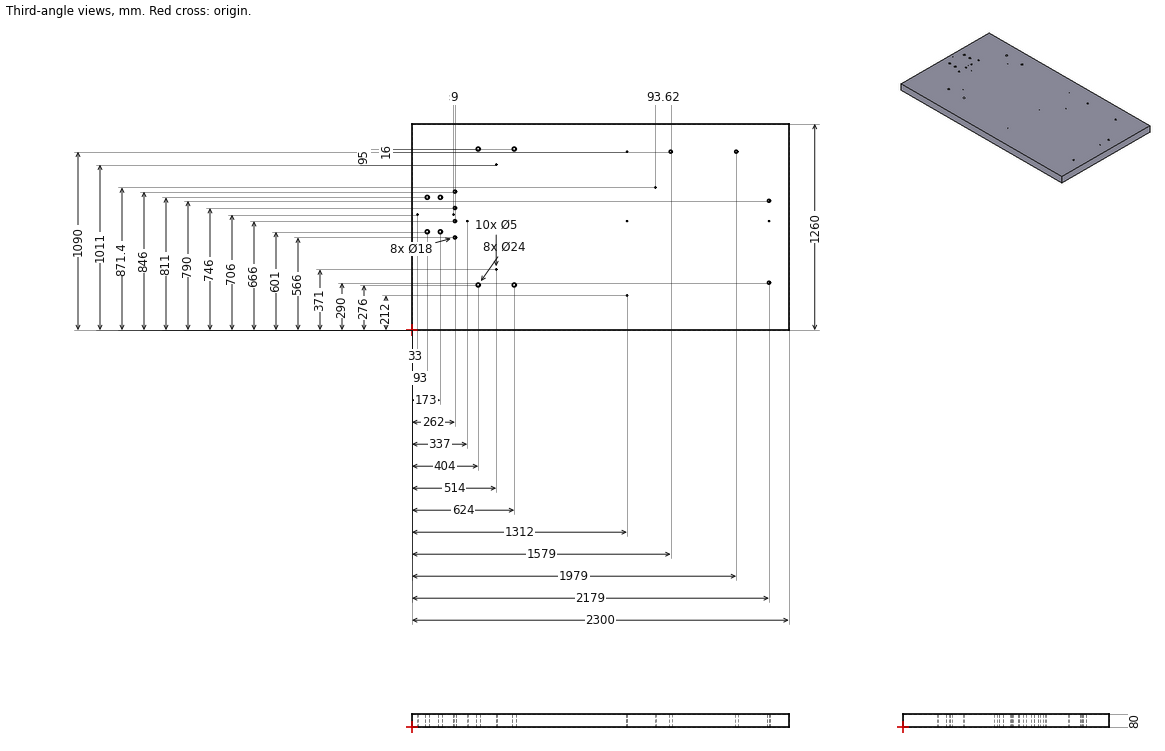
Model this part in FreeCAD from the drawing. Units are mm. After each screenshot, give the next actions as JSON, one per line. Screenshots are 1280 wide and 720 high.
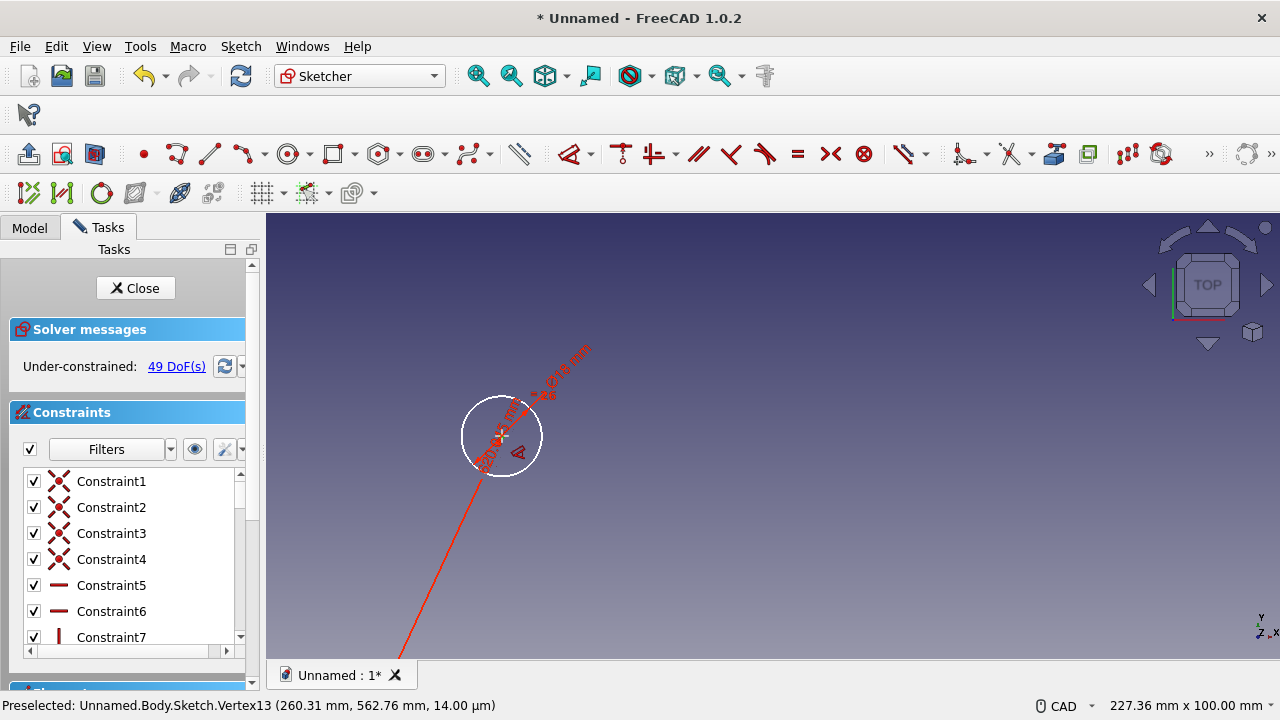
{"action": "scroll", "coordinate": [507, 452], "scroll_direction": "down", "scroll_amount": 15}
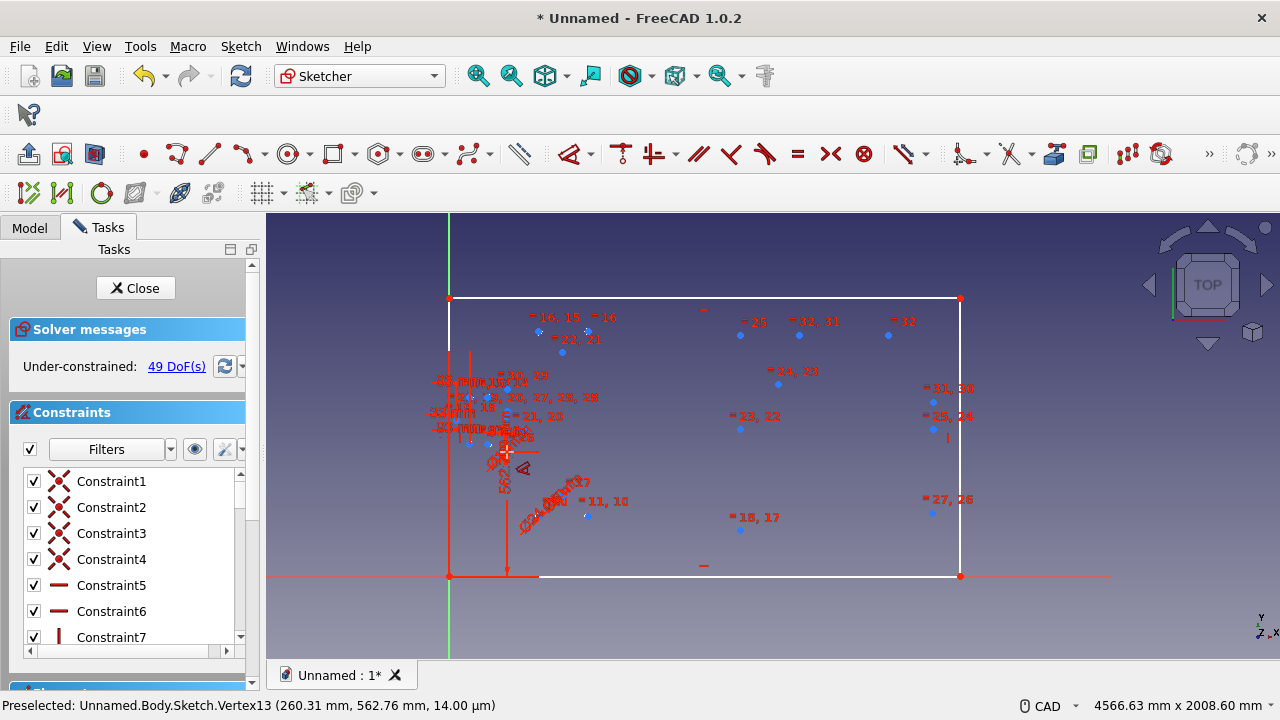
{"action": "scroll", "coordinate": [505, 420], "scroll_direction": "up", "scroll_amount": 15}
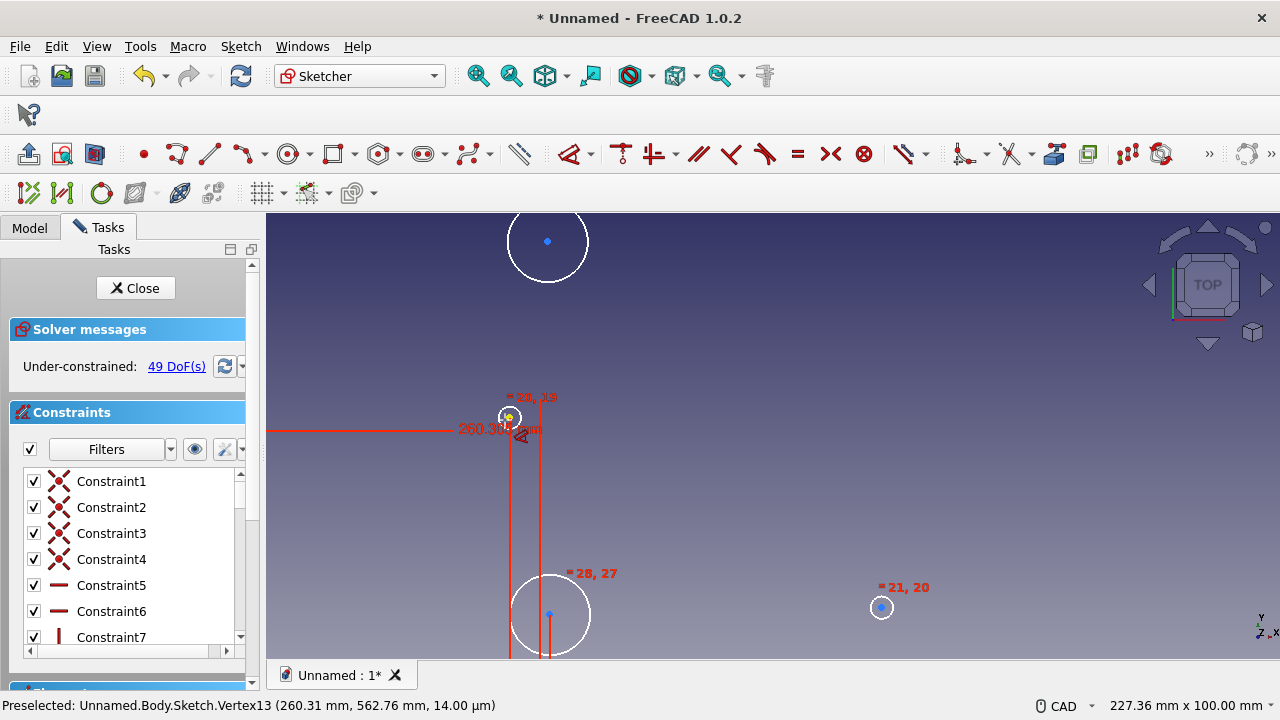
{"action": "left_click", "coordinate": [510, 418]}
{"action": "left_click", "coordinate": [525, 384]}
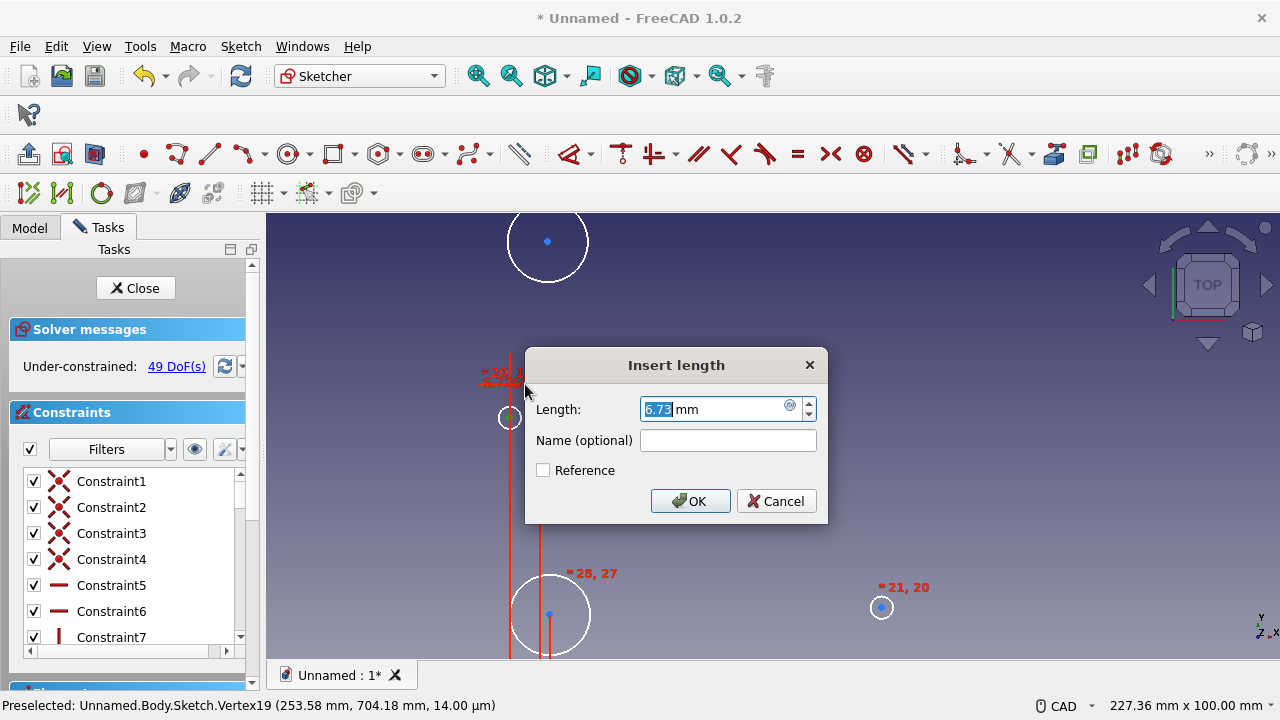
{"action": "type", "text": "9"}
{"action": "key", "text": "Return"}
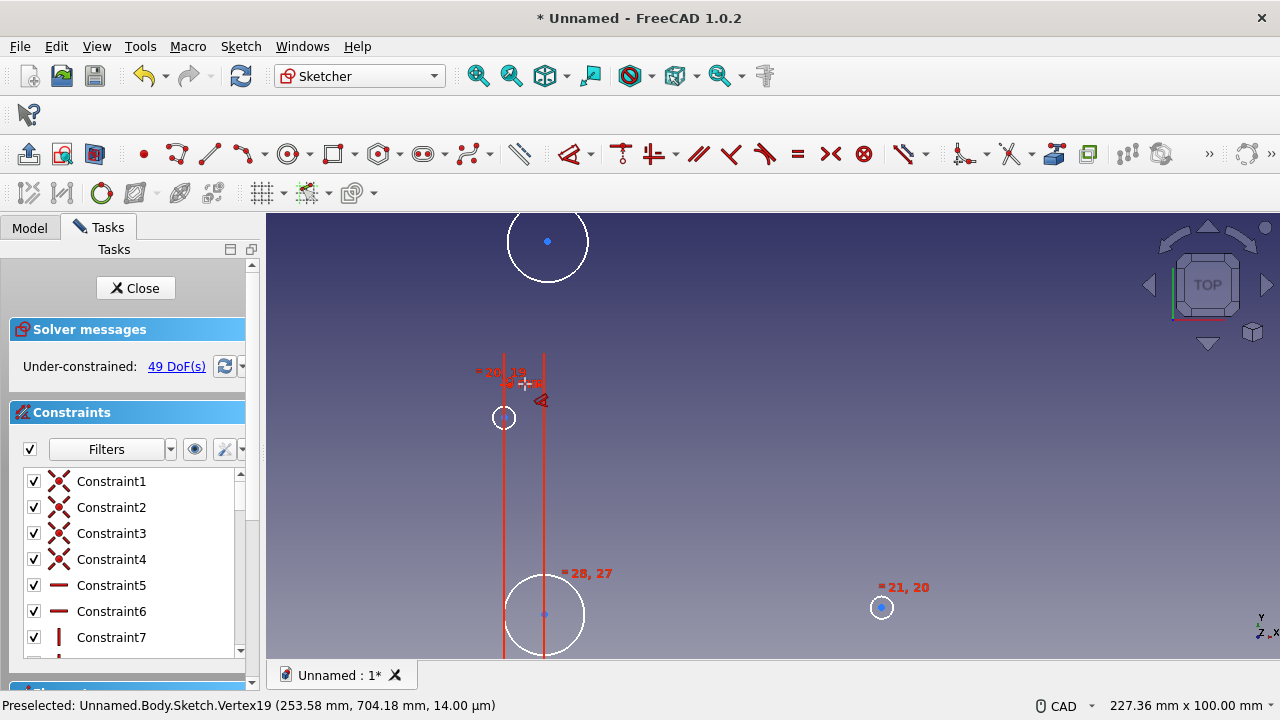
{"action": "left_click", "coordinate": [504, 418]}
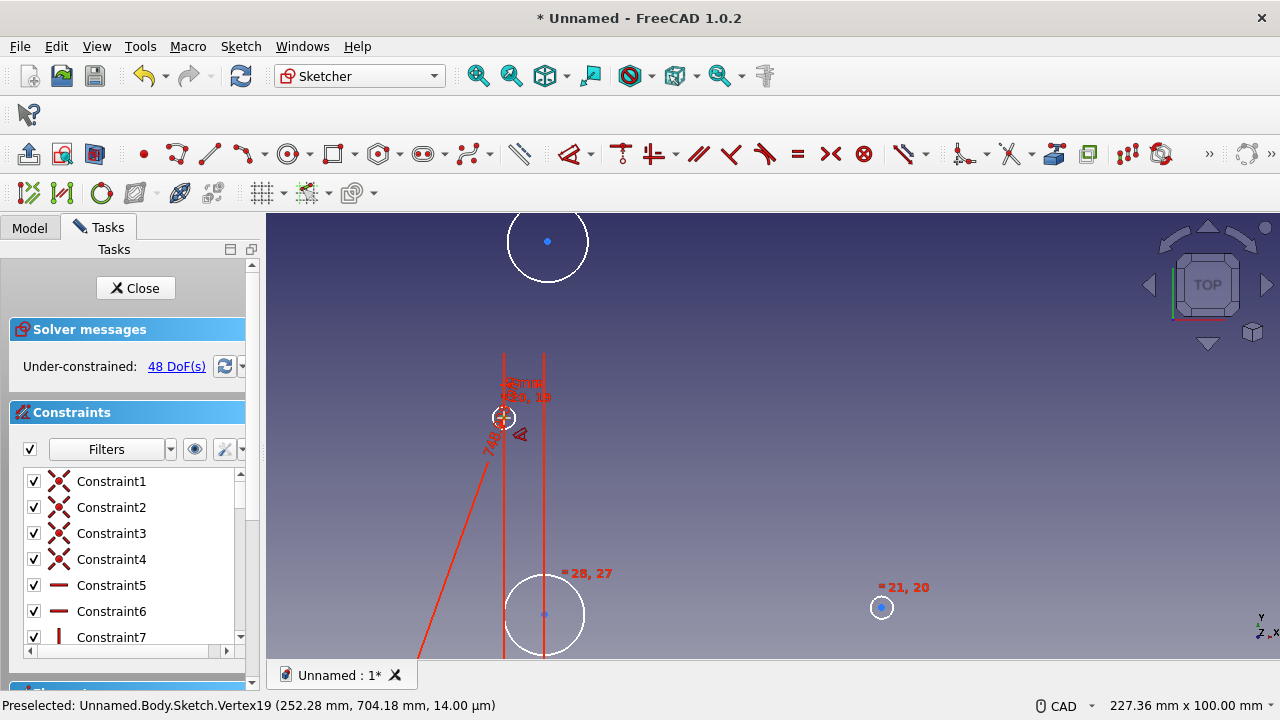
{"action": "left_click", "coordinate": [548, 242]}
{"action": "left_click", "coordinate": [526, 452]}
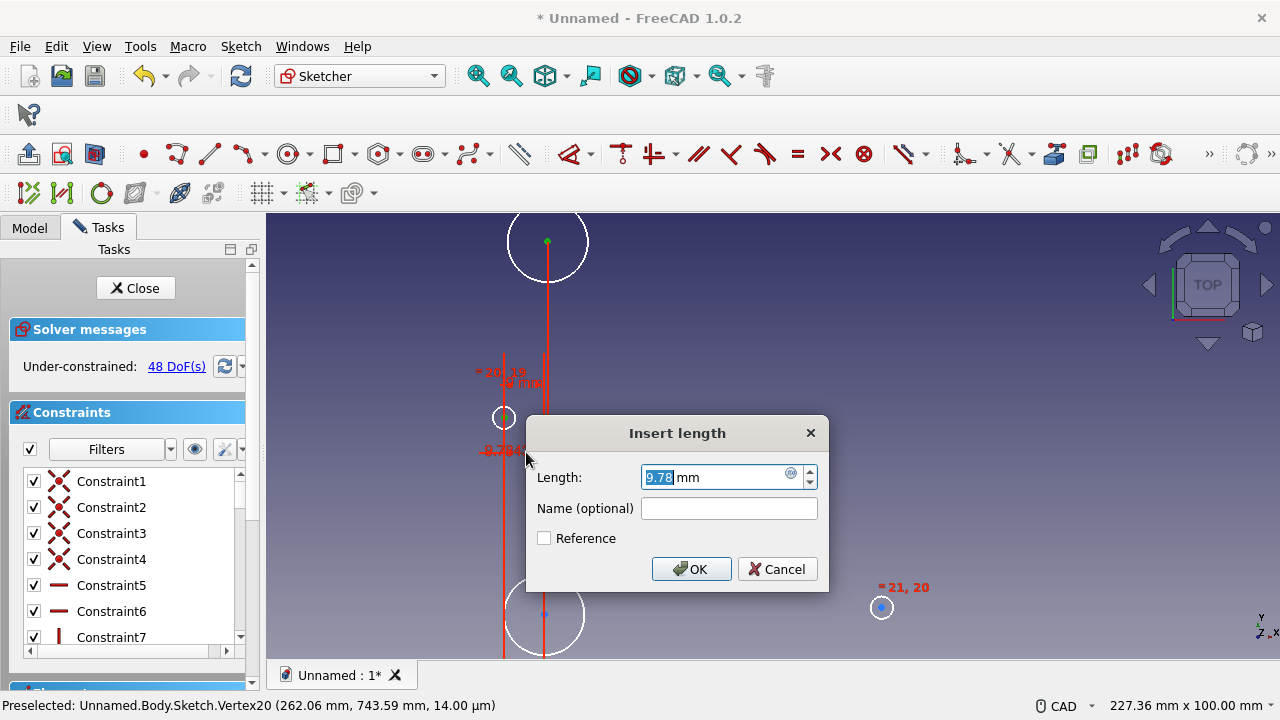
{"action": "type", "text": "9"}
{"action": "key", "text": "Return"}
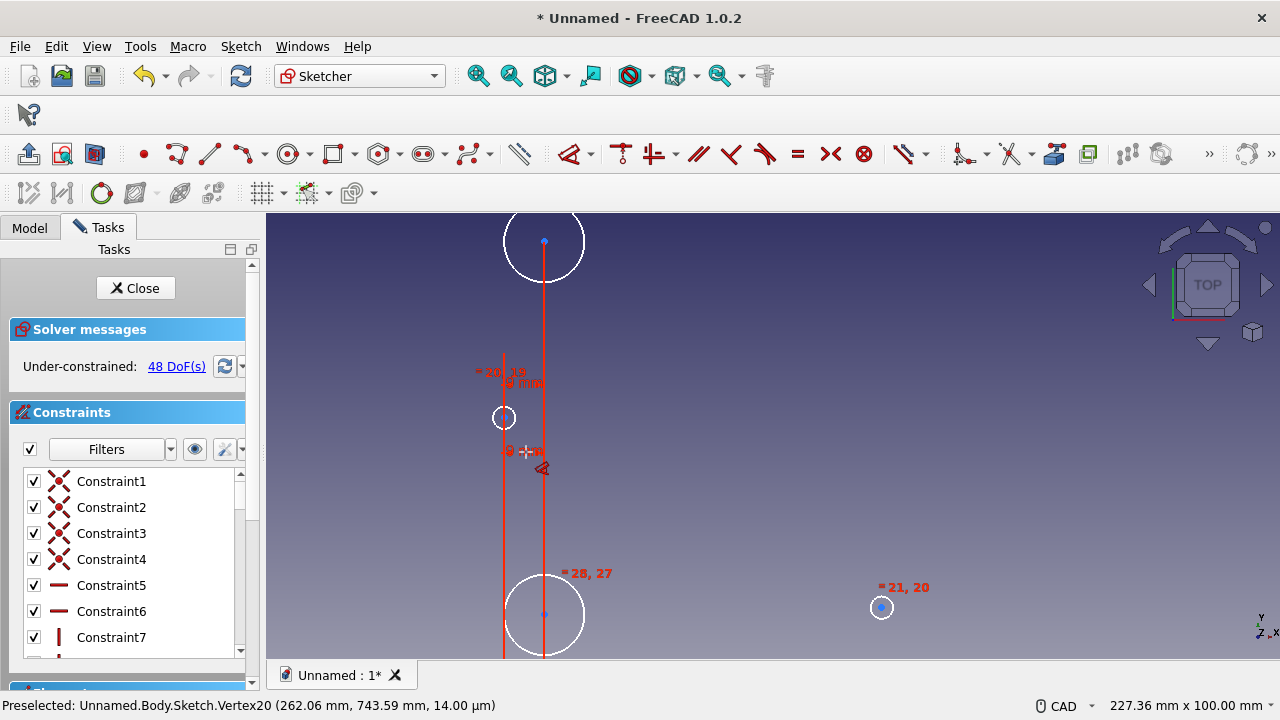
{"action": "left_click", "coordinate": [504, 418]}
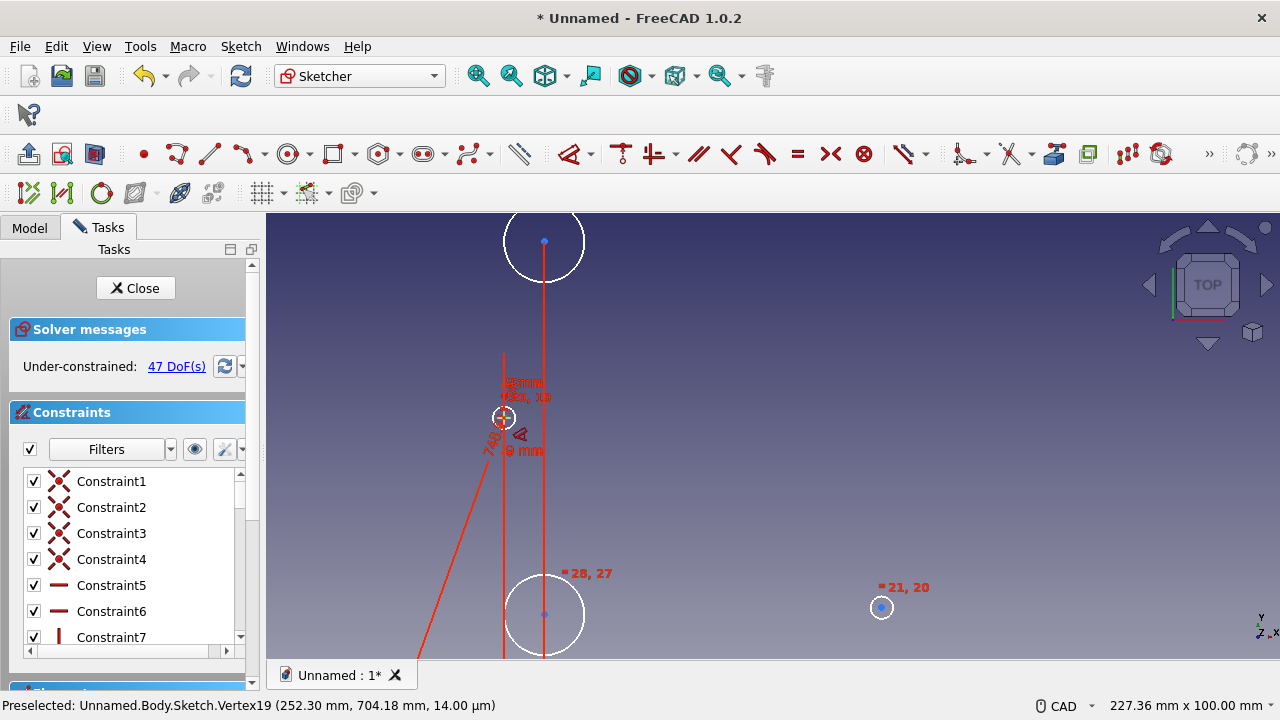
{"action": "scroll", "coordinate": [505, 420], "scroll_direction": "down", "scroll_amount": 15}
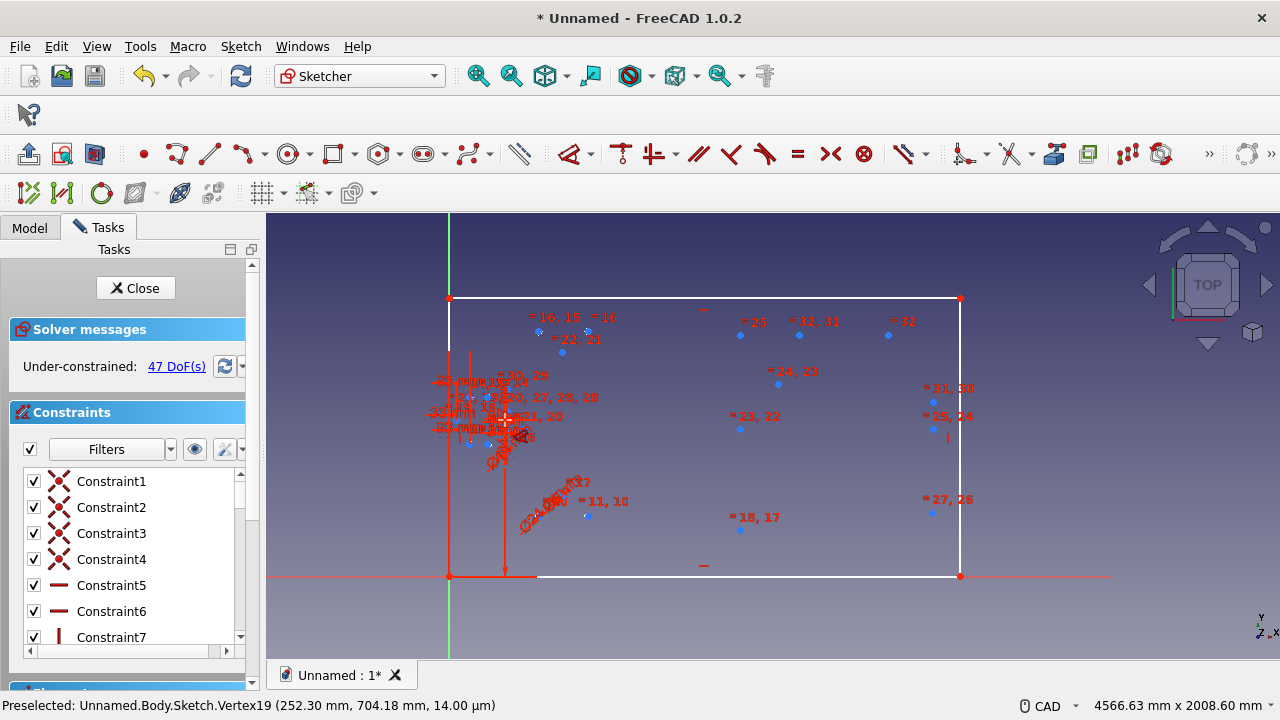
{"action": "scroll", "coordinate": [507, 390], "scroll_direction": "up", "scroll_amount": 15}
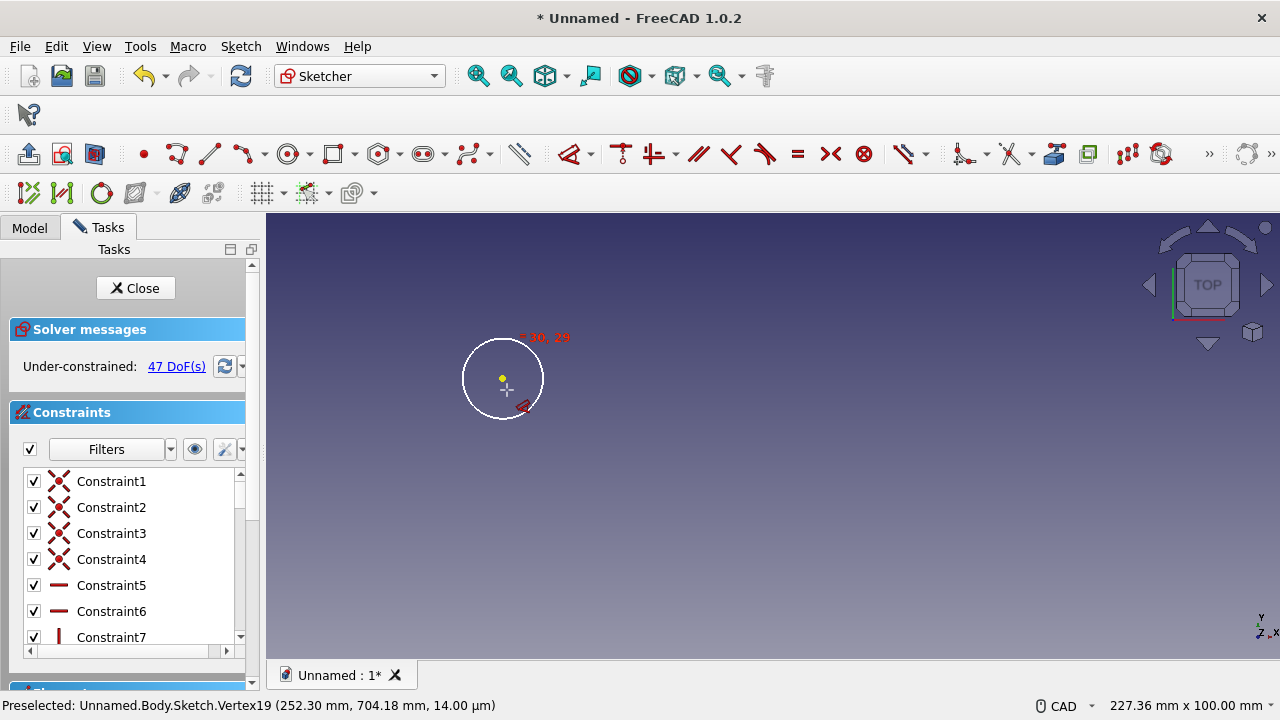
{"action": "left_click", "coordinate": [503, 379]}
{"action": "left_click", "coordinate": [484, 321]}